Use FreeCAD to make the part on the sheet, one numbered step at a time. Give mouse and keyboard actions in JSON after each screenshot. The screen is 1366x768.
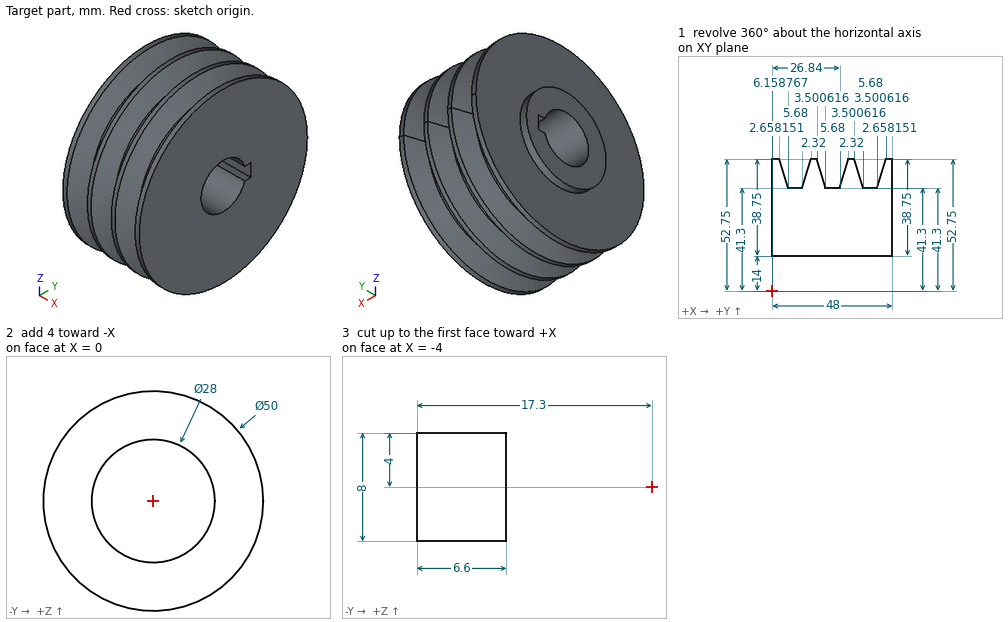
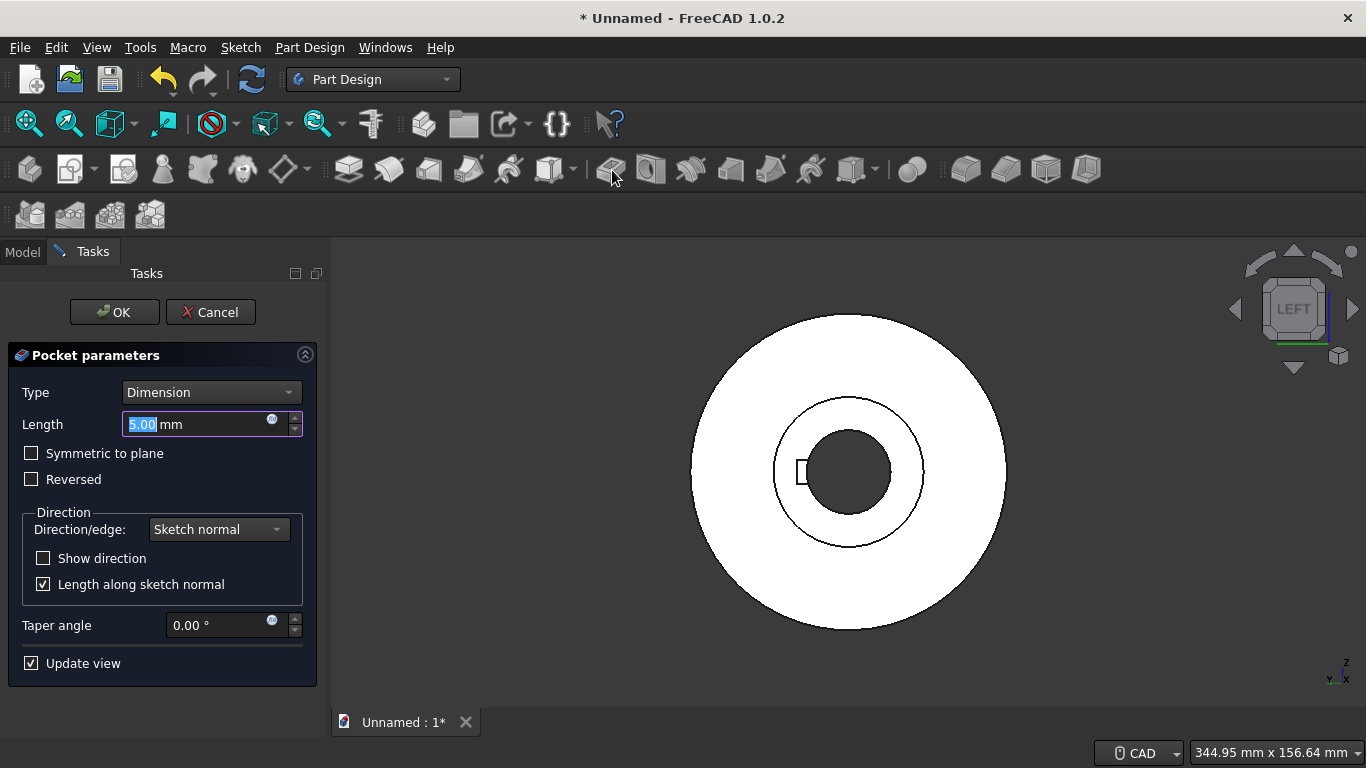
{"action": "left_click", "coordinate": [212, 392]}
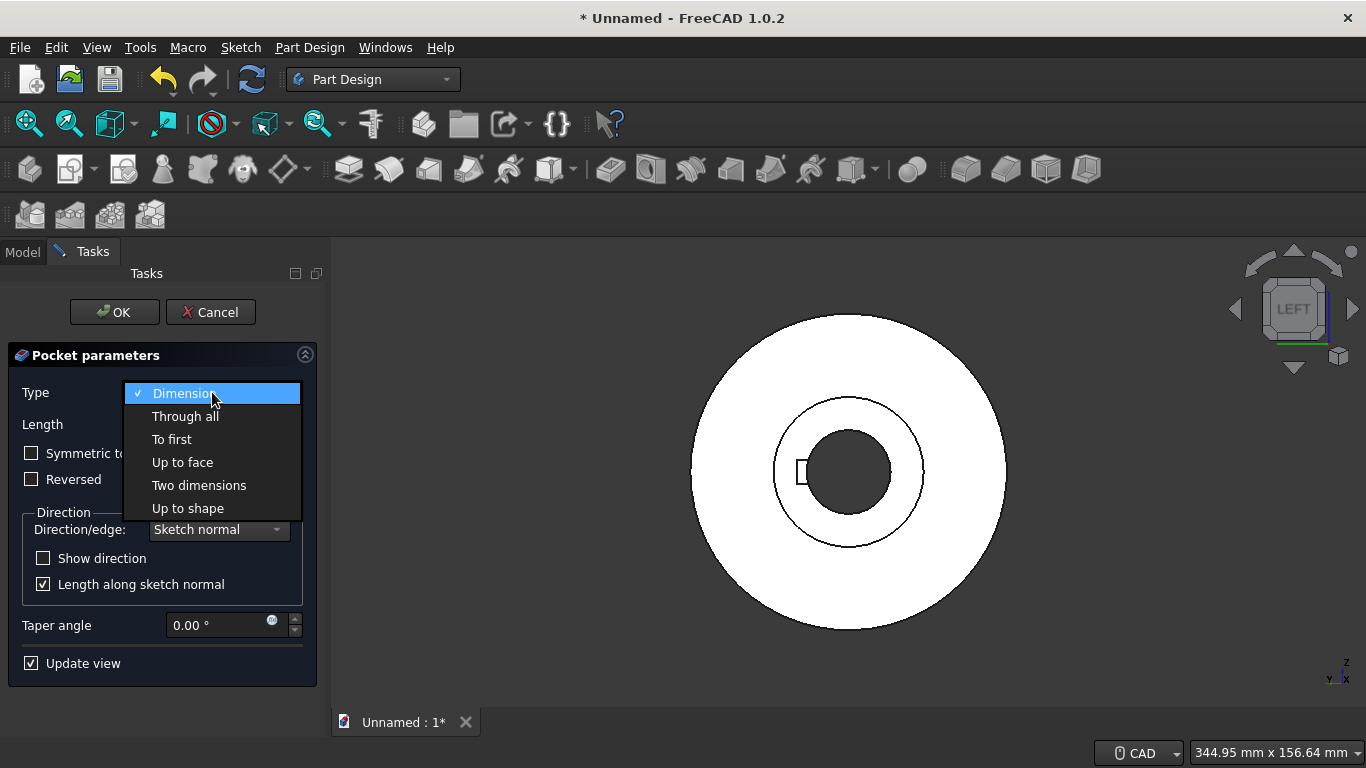
{"action": "left_click", "coordinate": [212, 440]}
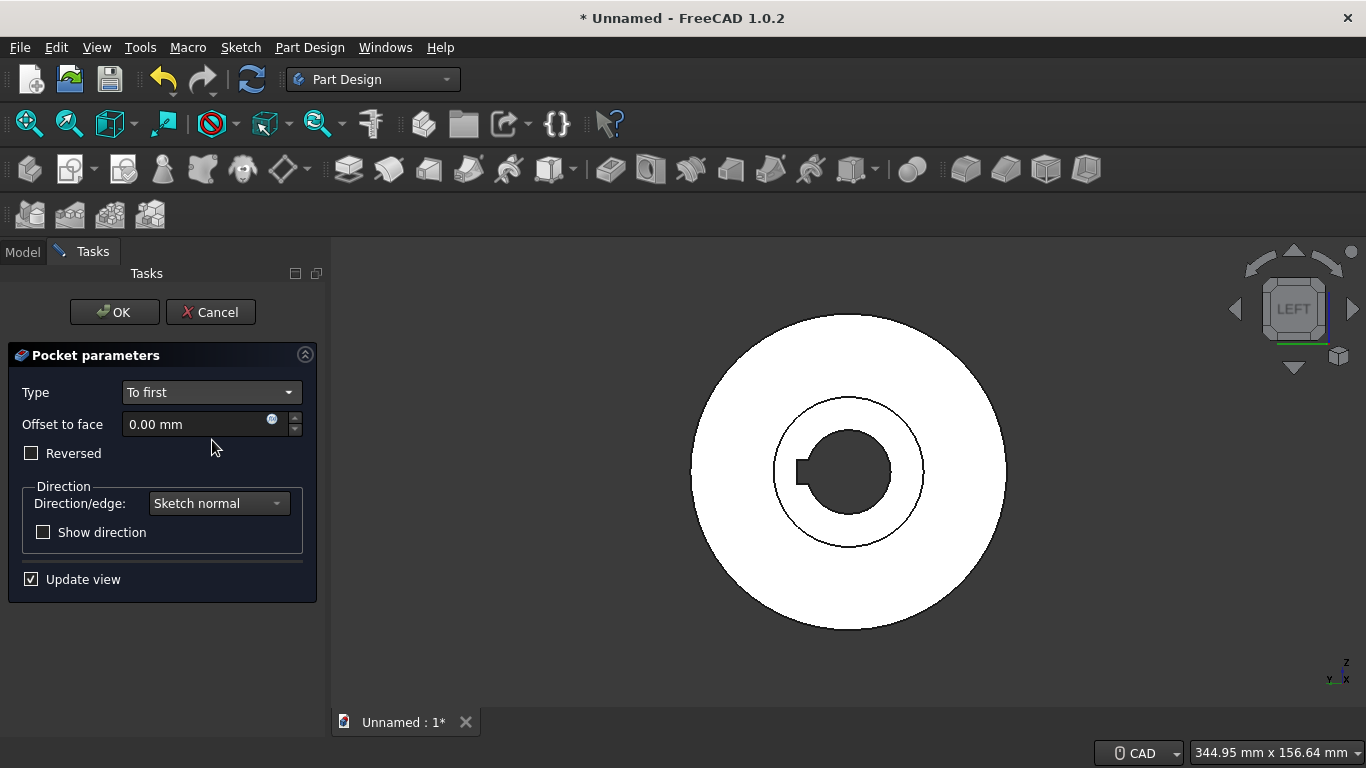
{"action": "left_click", "coordinate": [115, 312]}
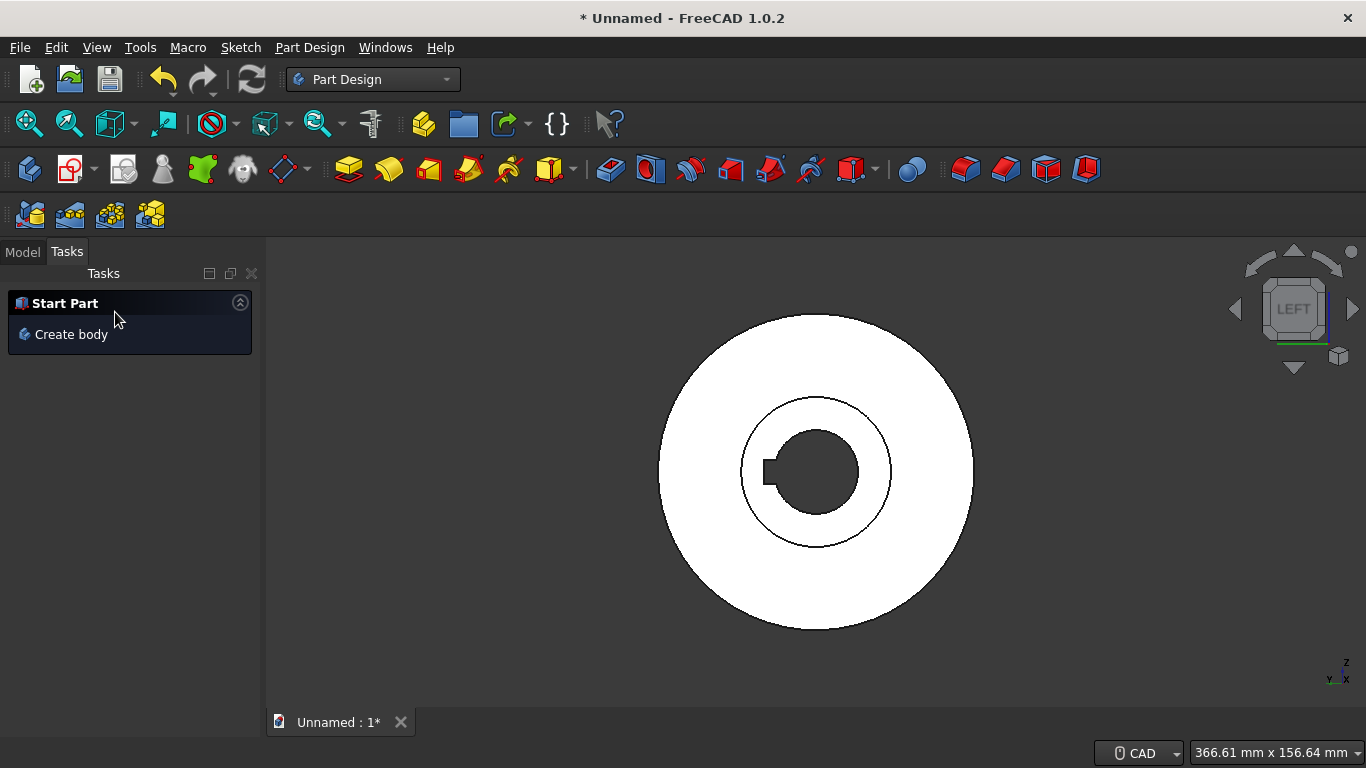
{"action": "key", "text": "0"}